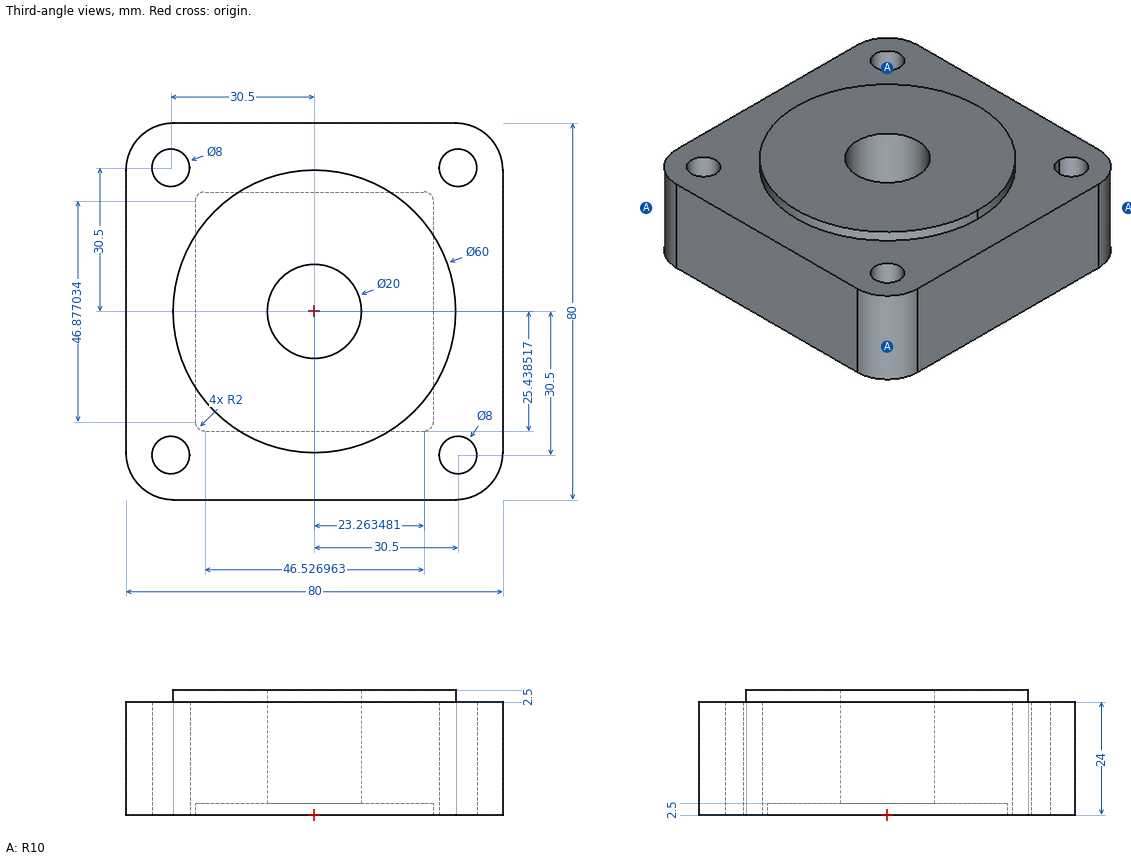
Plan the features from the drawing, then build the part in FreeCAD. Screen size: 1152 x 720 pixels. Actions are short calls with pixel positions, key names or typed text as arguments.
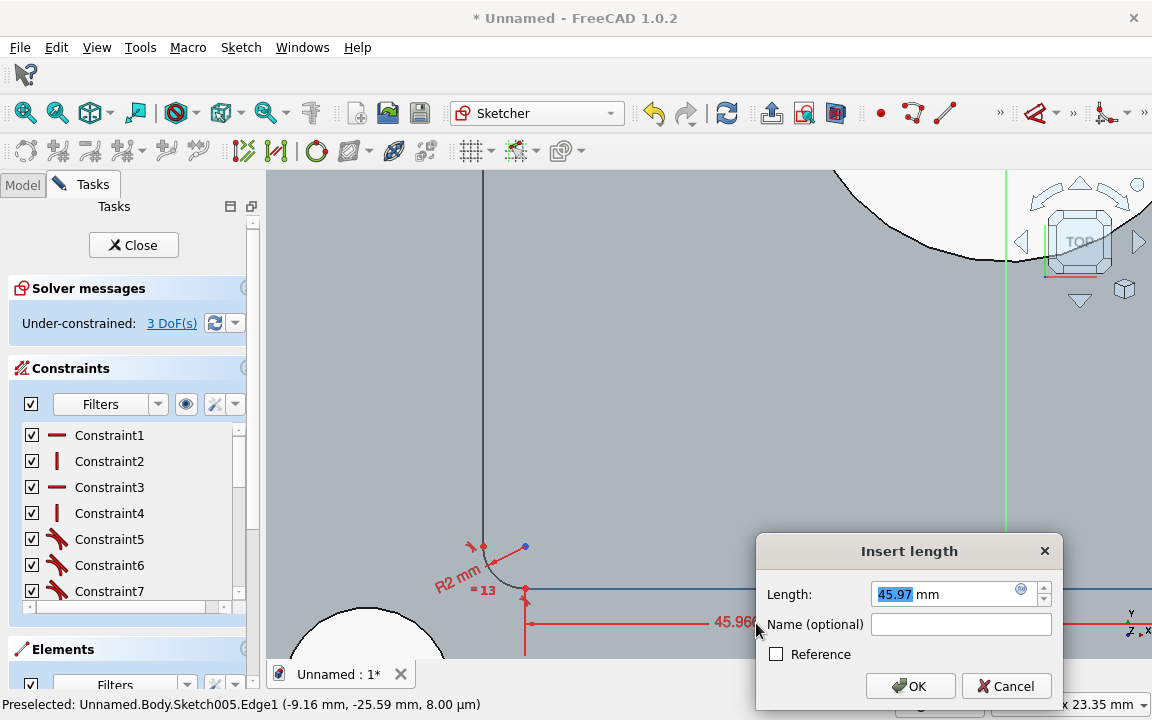
text(46.526963)
key(Return)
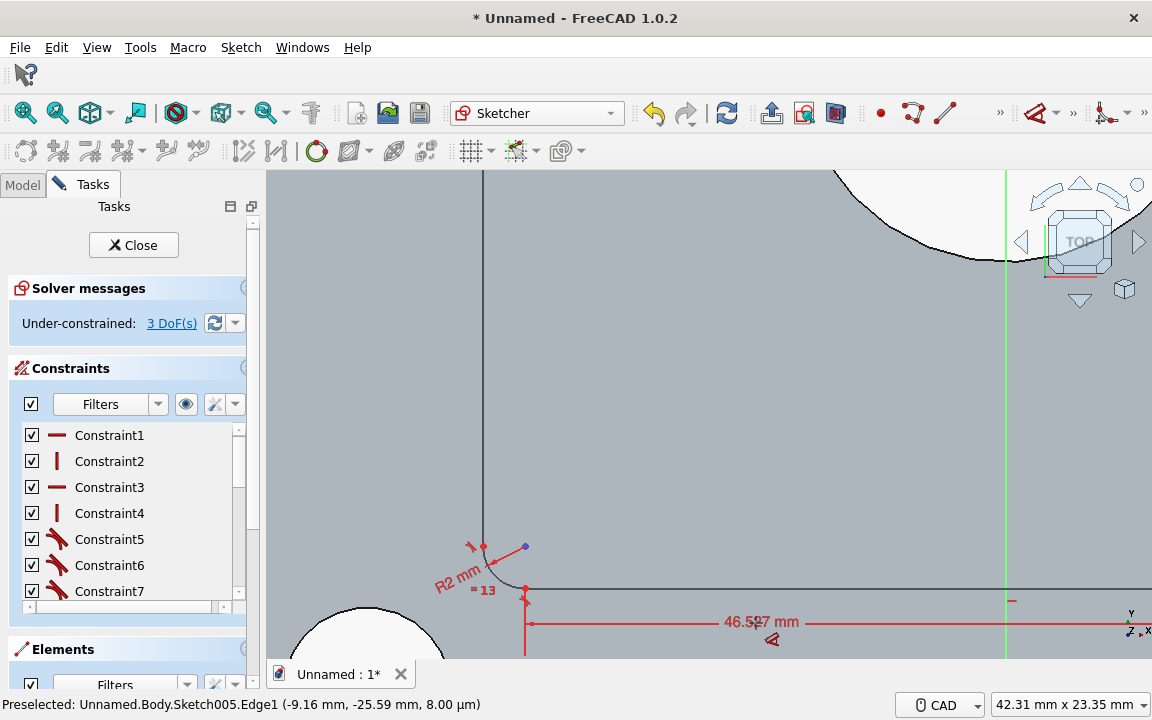
click(483, 251)
click(449, 372)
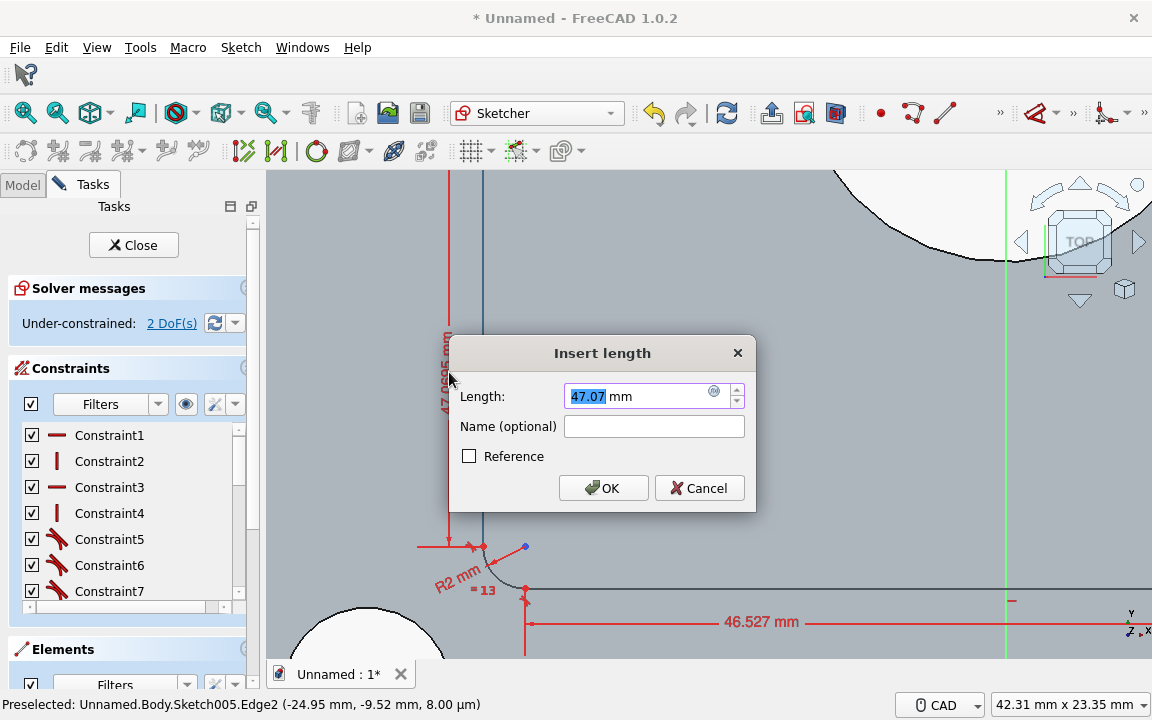
text(46.877034)
key(Return)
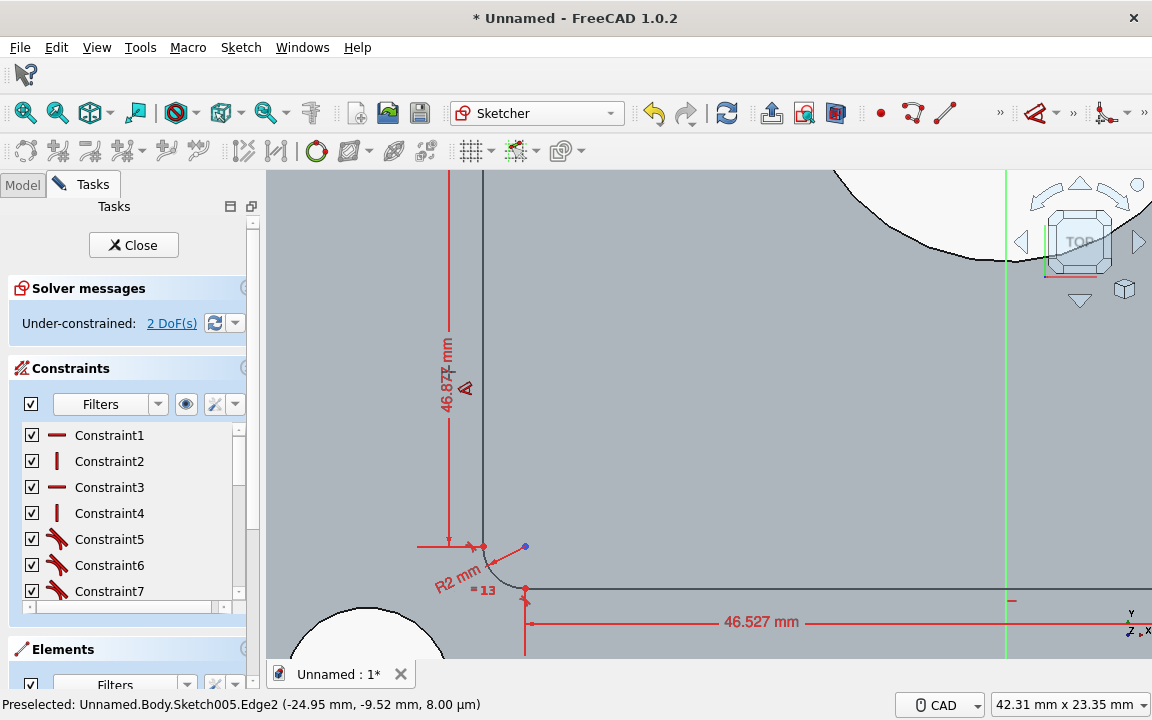
scroll(483, 570, down, 6)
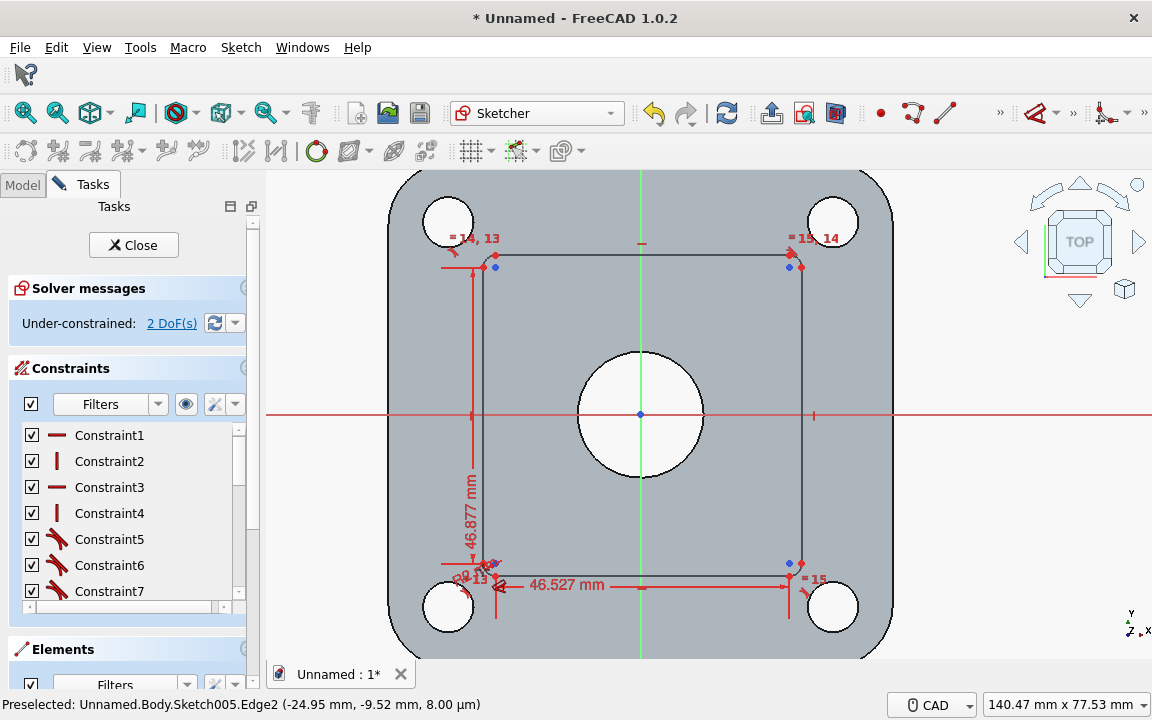
click(789, 576)
click(715, 610)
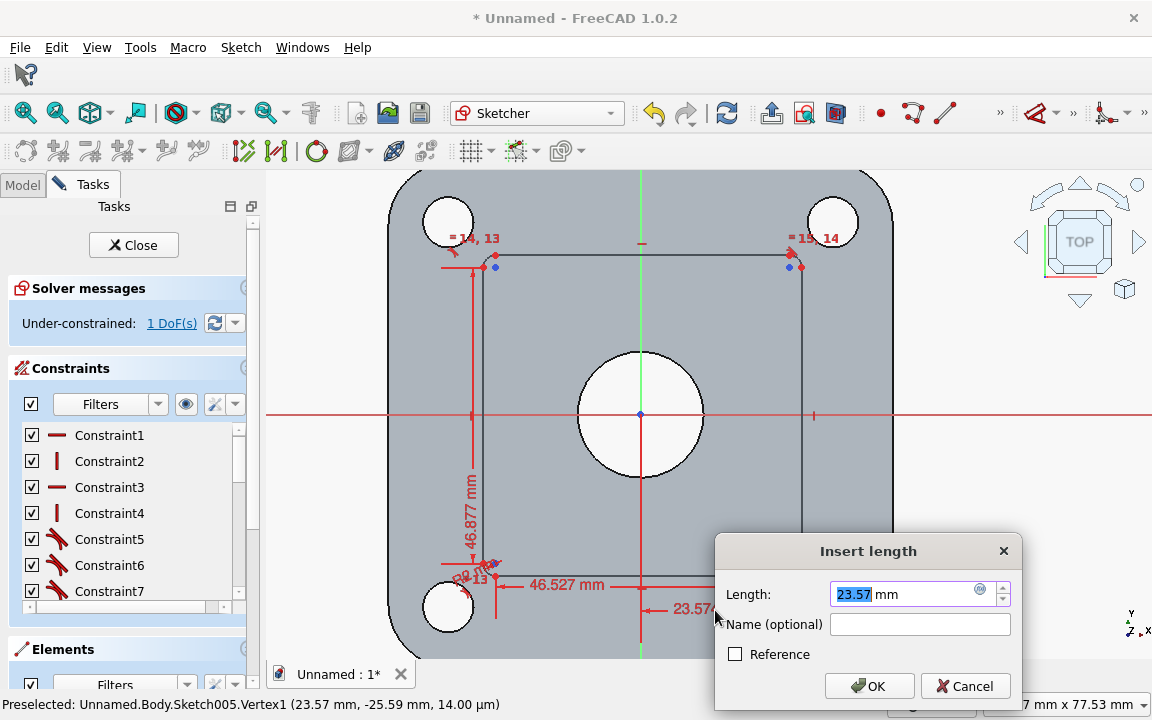
text(23.263481)
key(Return)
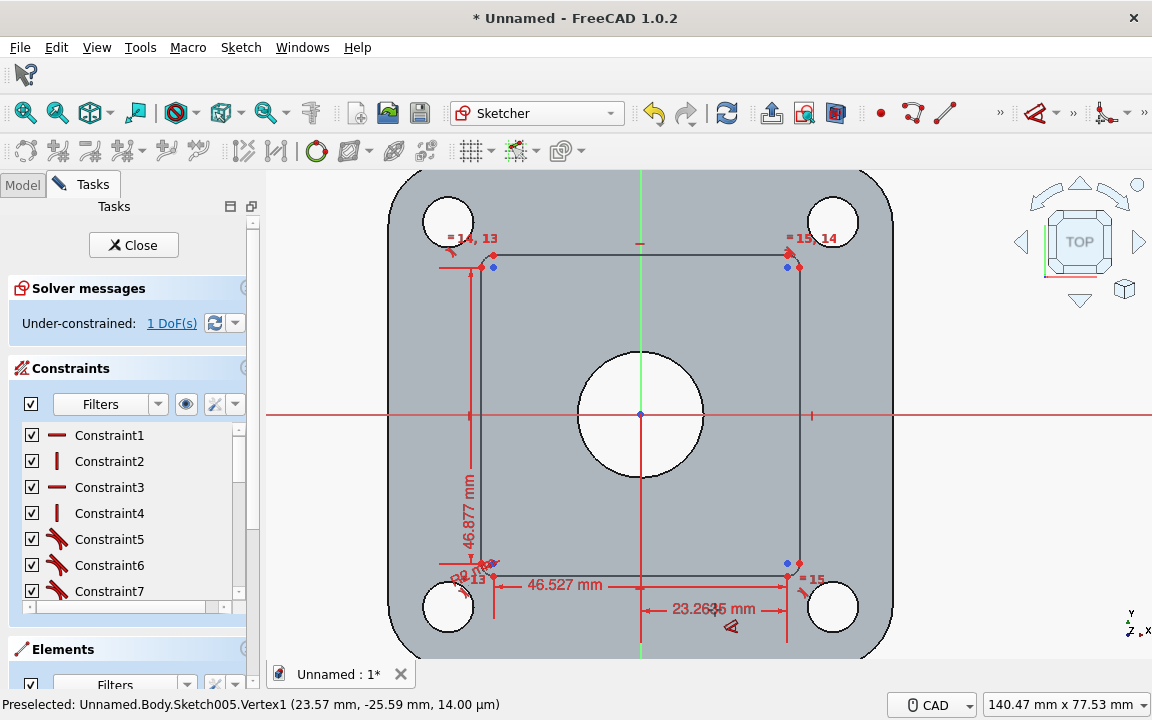
click(787, 576)
click(821, 495)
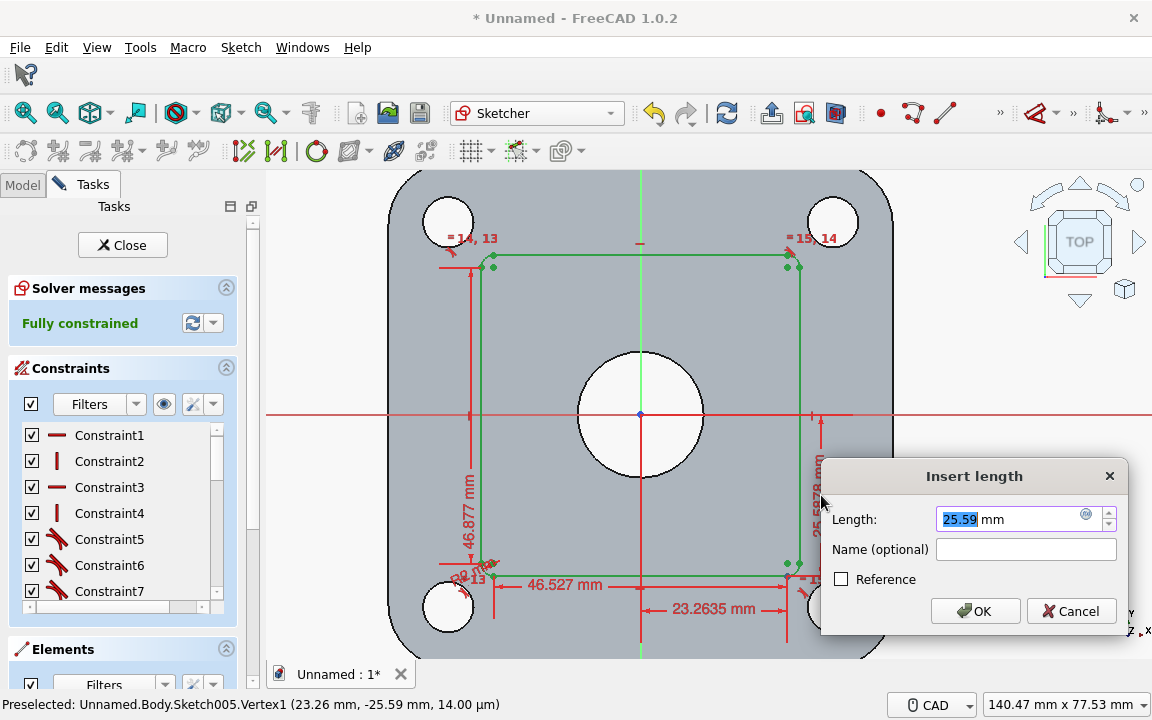
text(25.438517)
key(Return)
key(Escape)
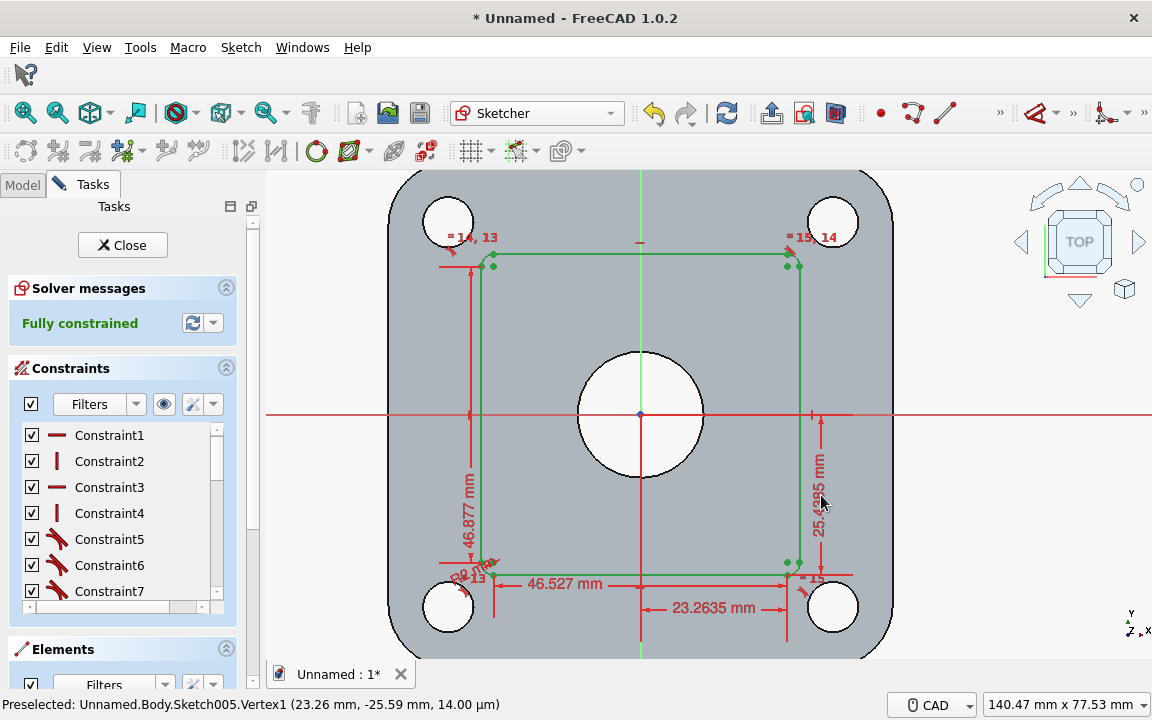
click(123, 245)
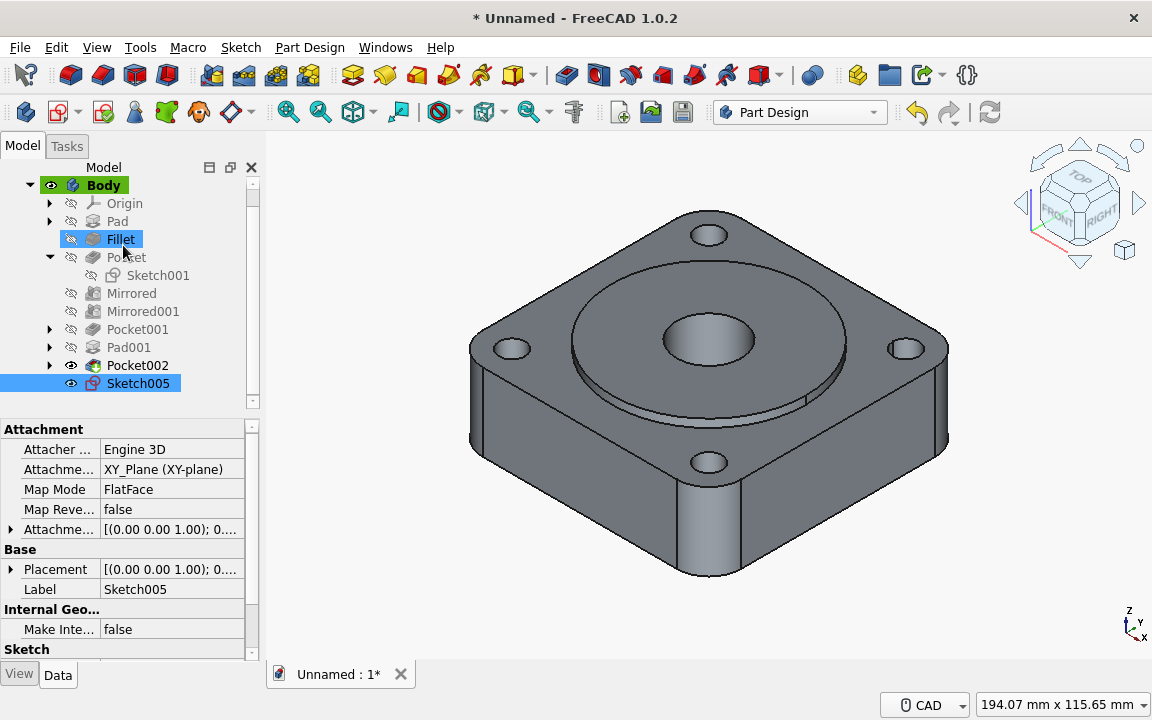
click(568, 76)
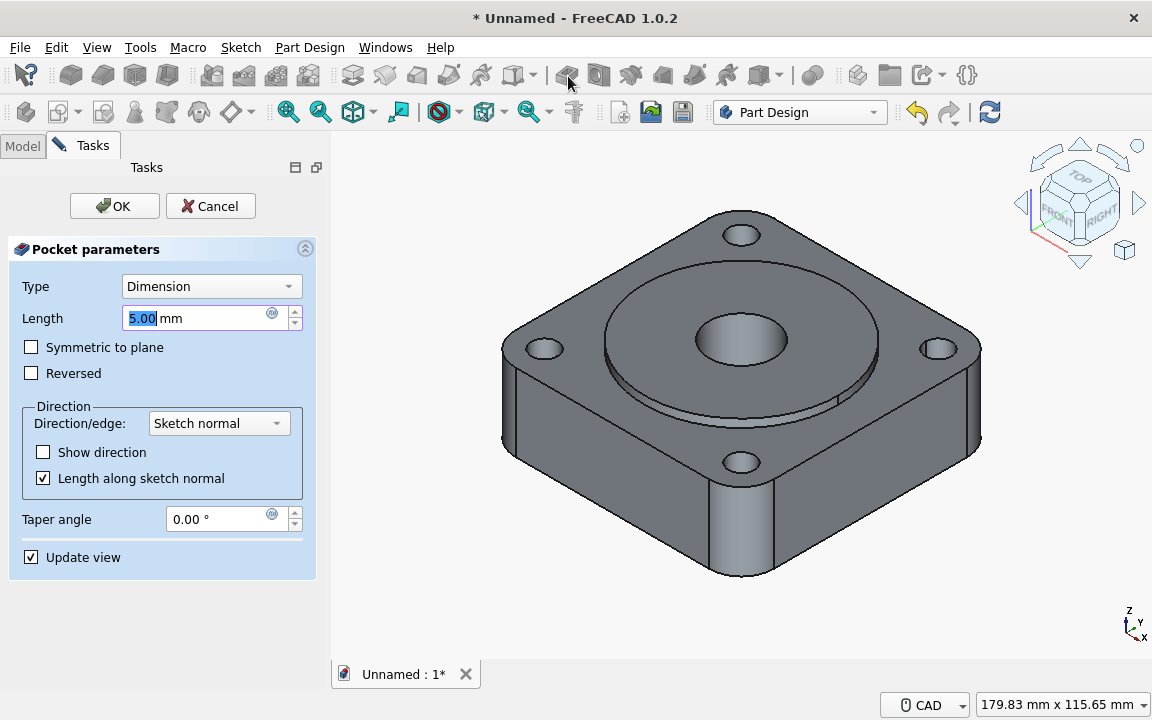
text(2.5)
key(Tab)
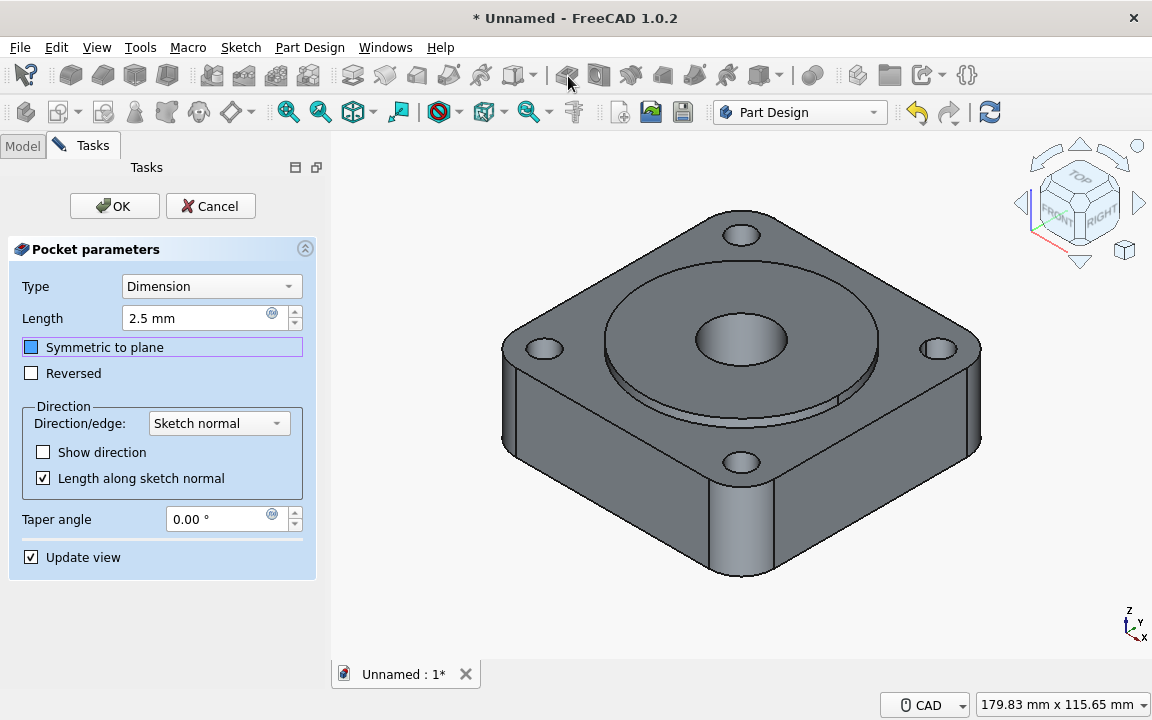
click(30, 373)